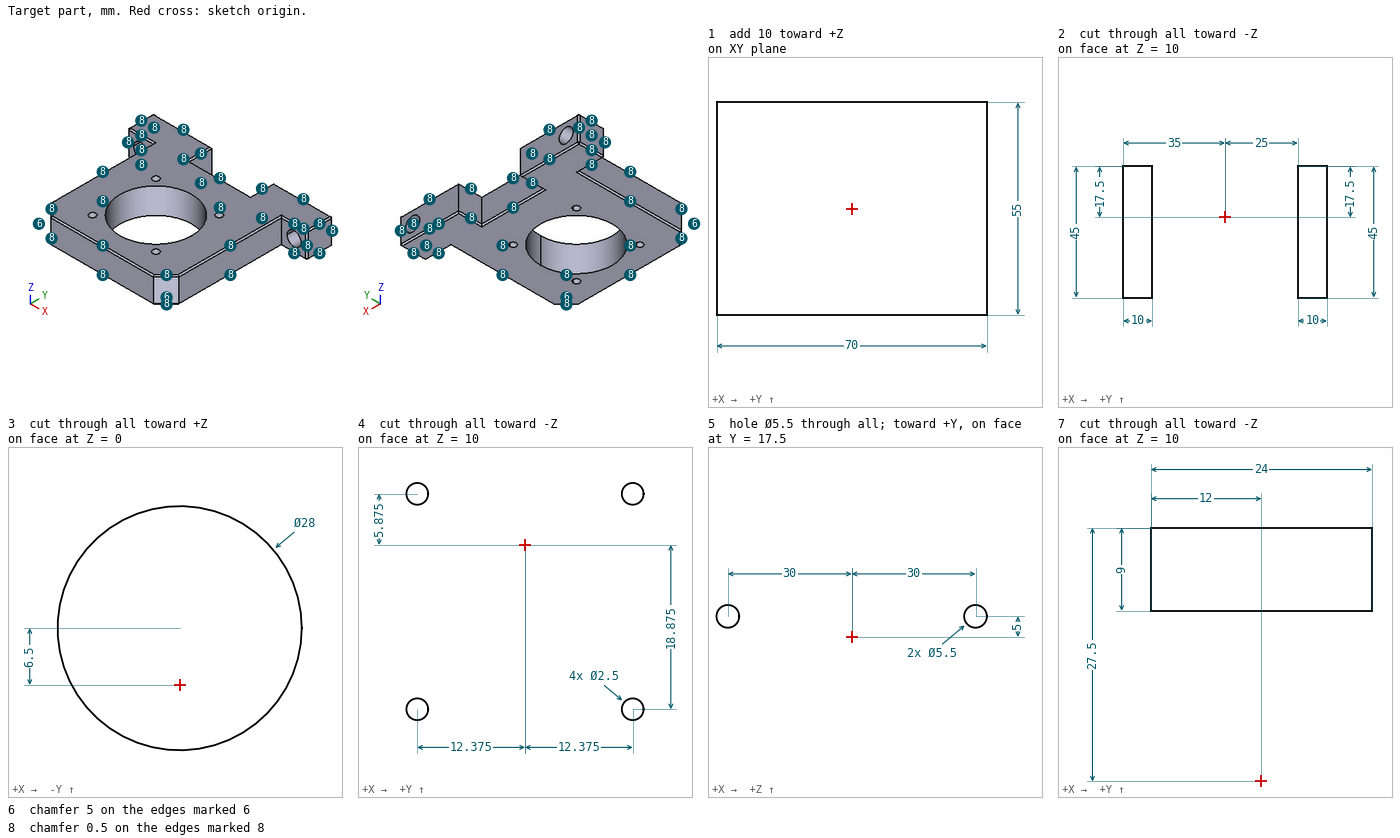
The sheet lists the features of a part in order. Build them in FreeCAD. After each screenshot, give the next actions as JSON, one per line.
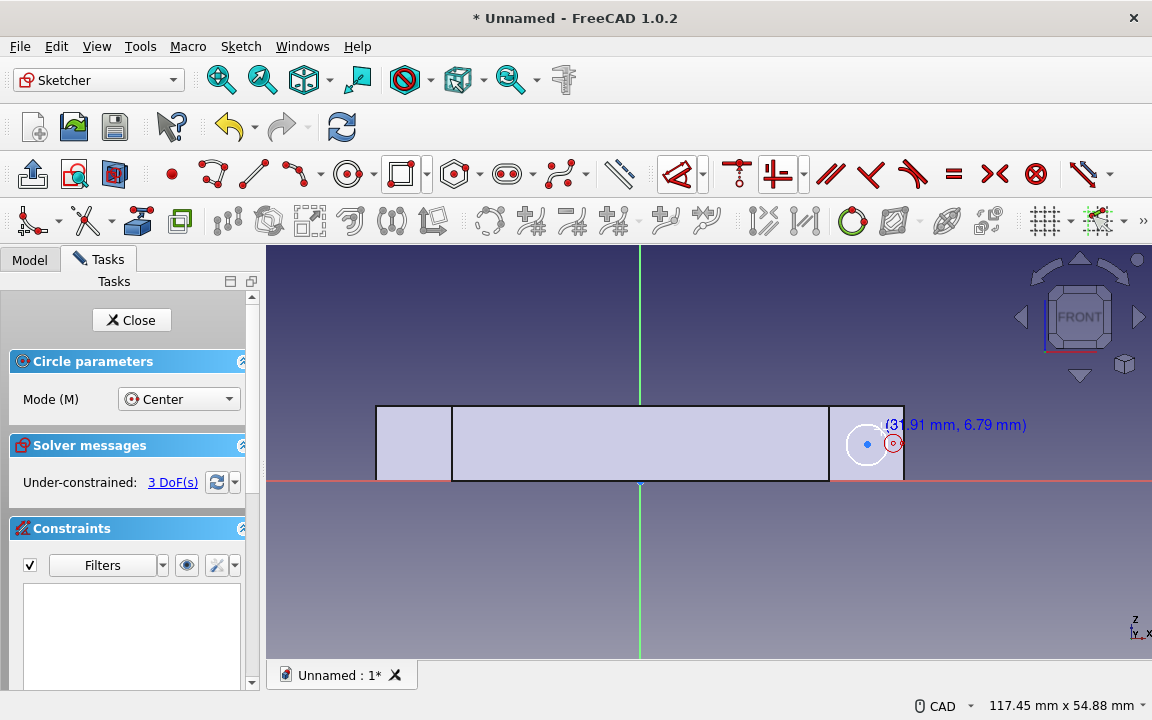
{"action": "left_click", "coordinate": [414, 444]}
{"action": "left_click", "coordinate": [429, 429]}
{"action": "key", "text": "Escape"}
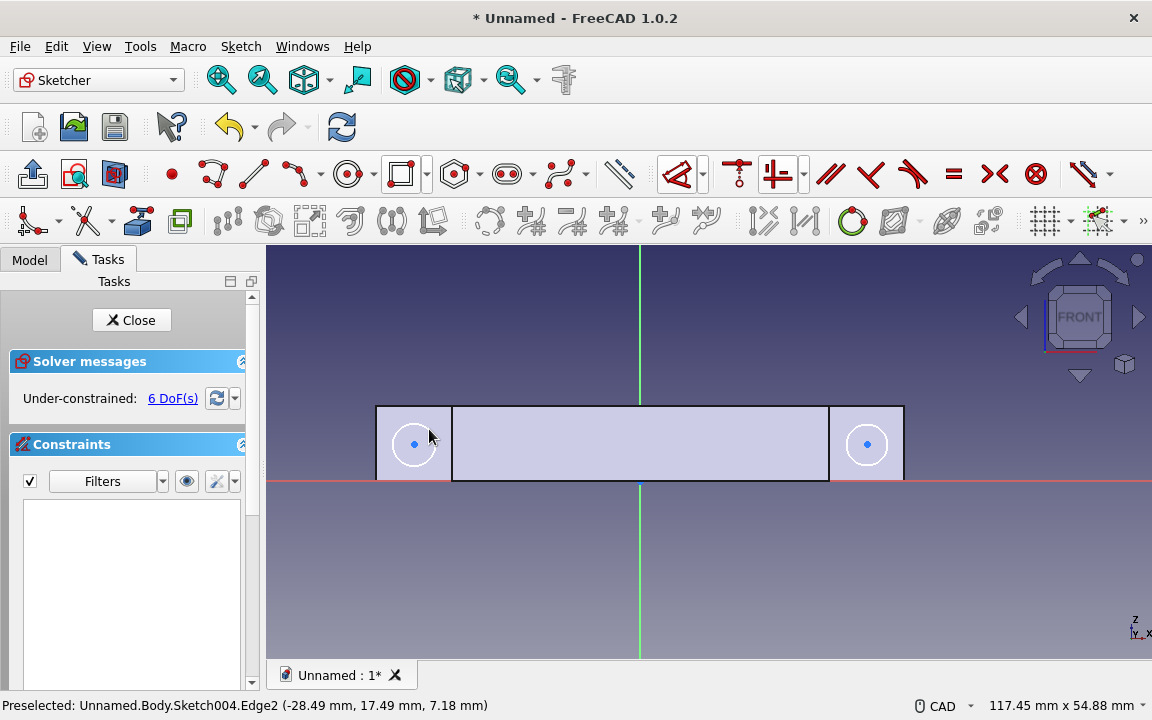
{"action": "left_click", "coordinate": [881, 430]}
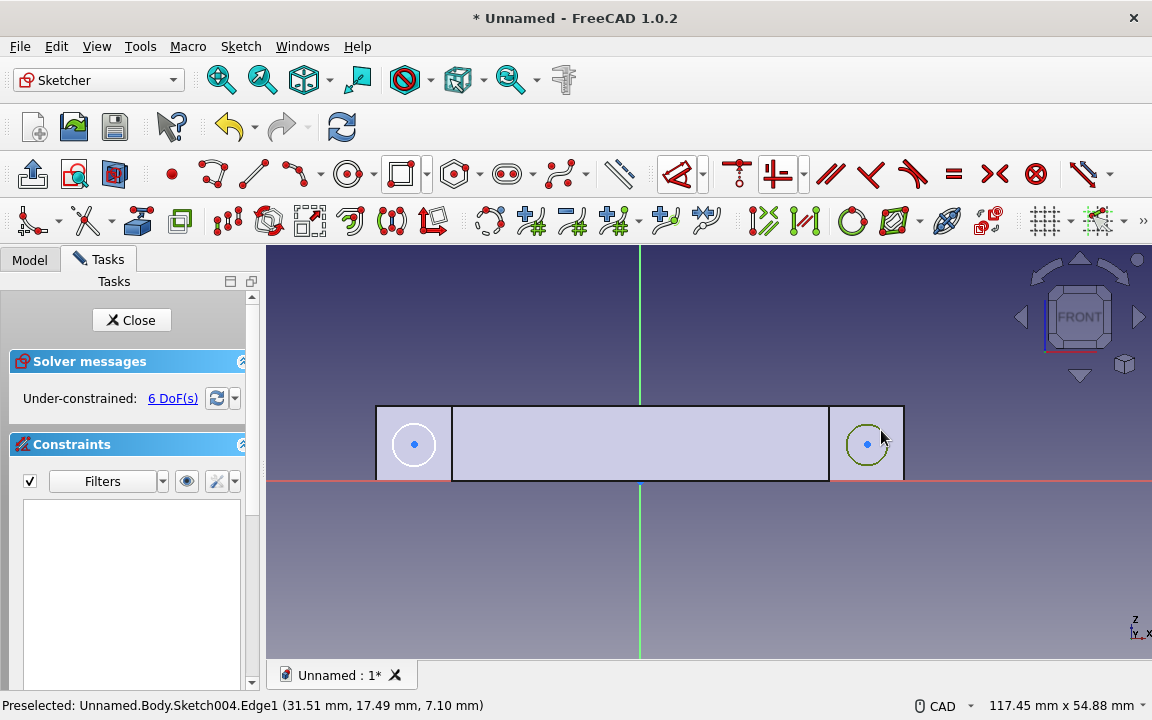
{"action": "left_click", "coordinate": [429, 430]}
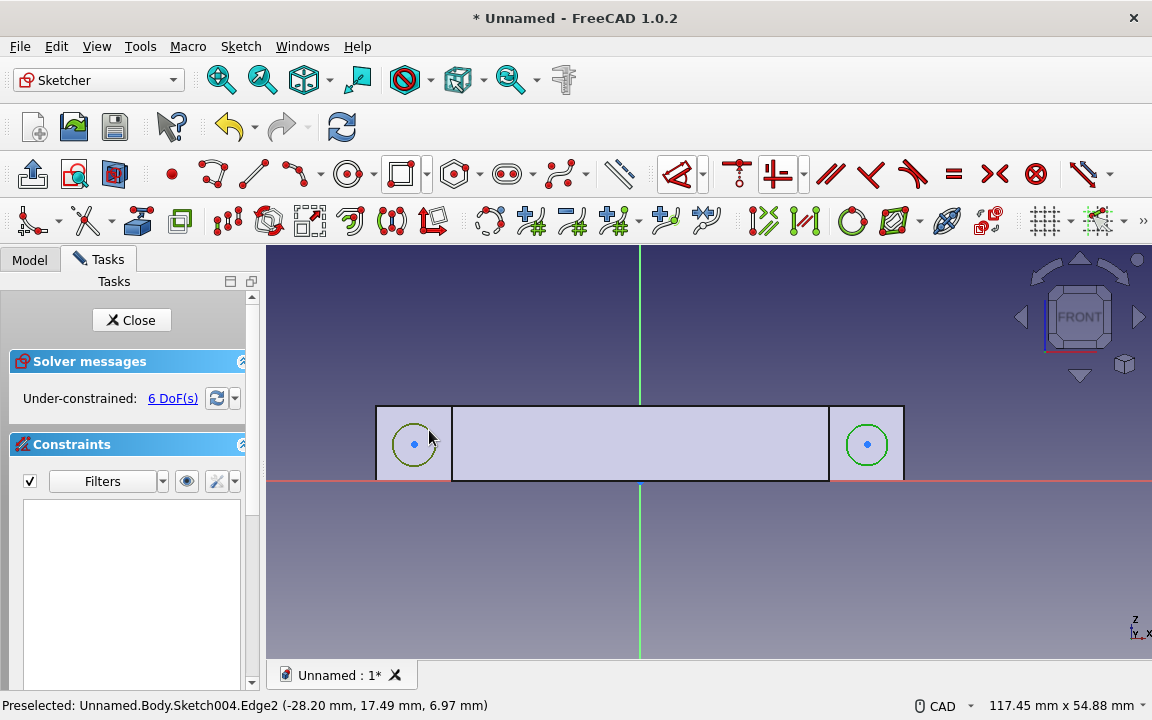
{"action": "left_click", "coordinate": [954, 174]}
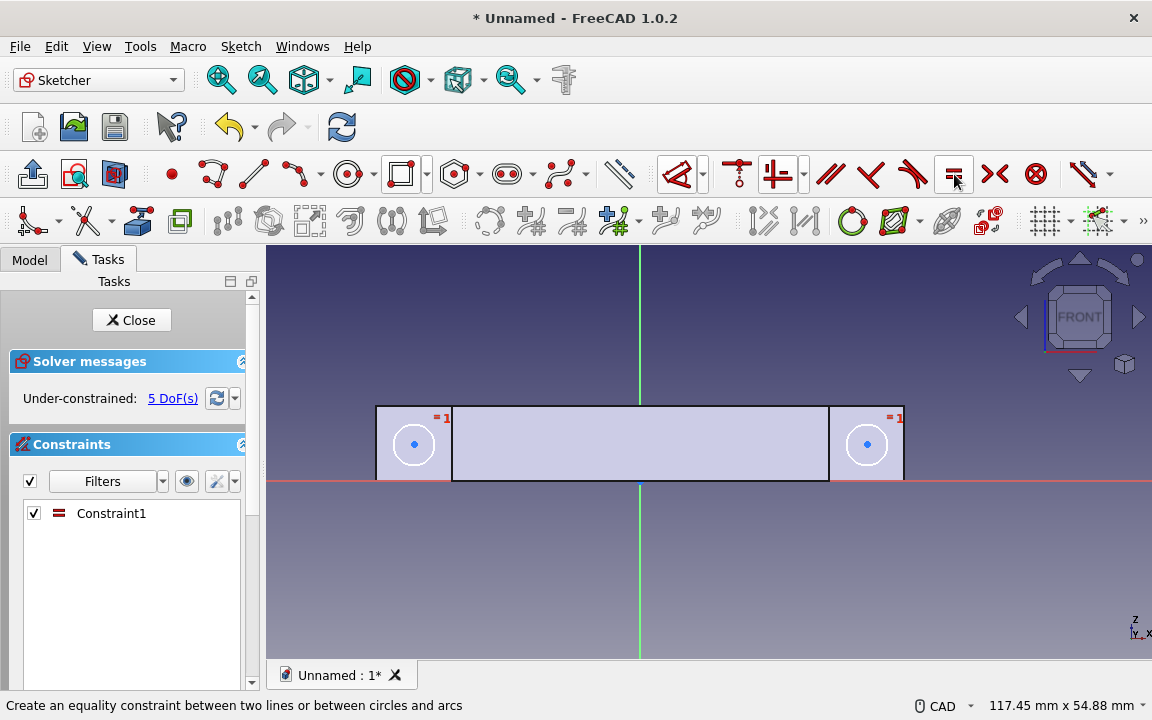
{"action": "left_click", "coordinate": [867, 445]}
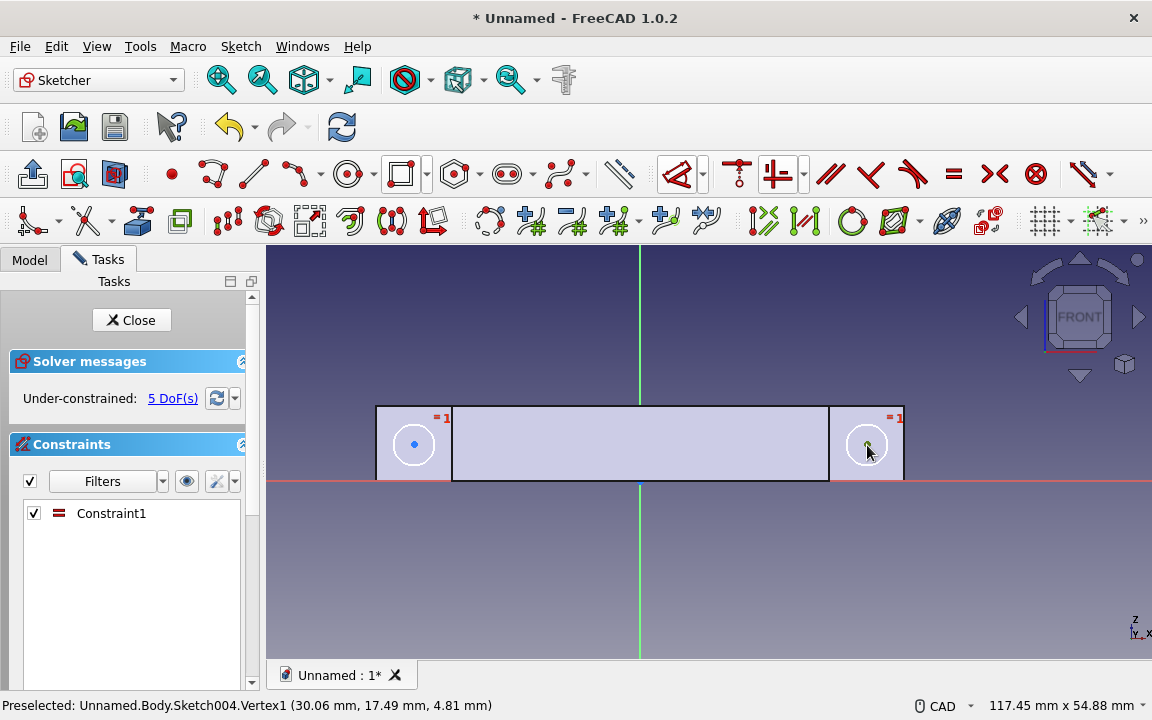
{"action": "left_click", "coordinate": [414, 445]}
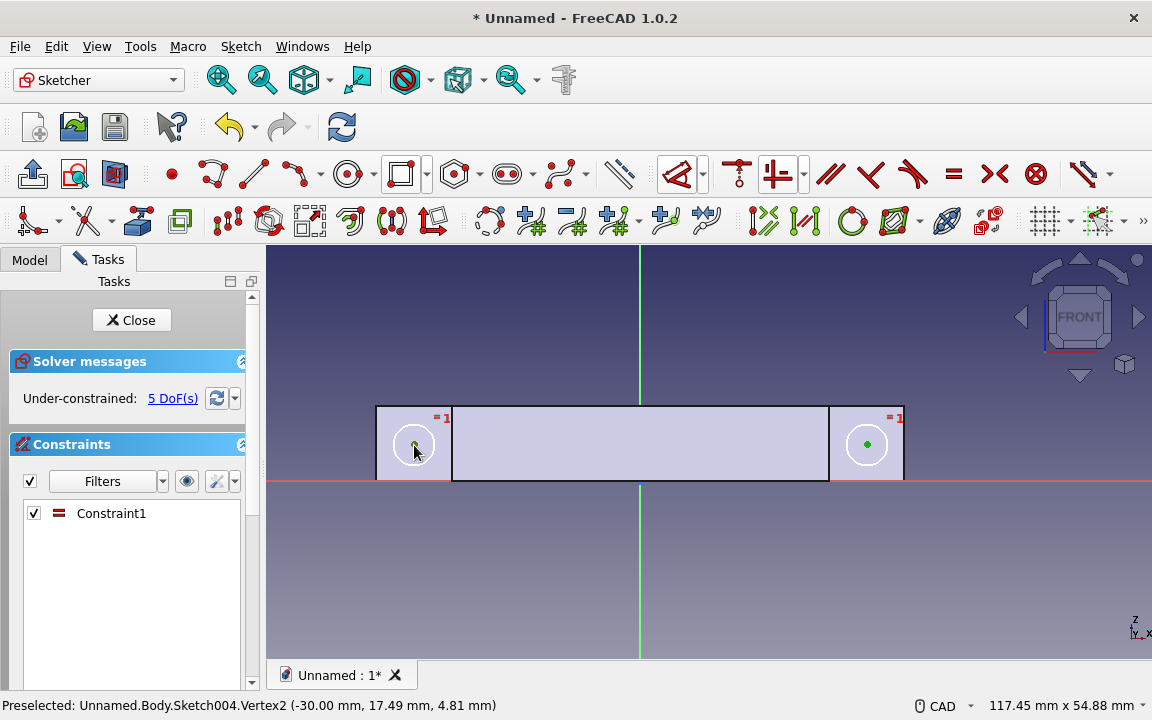
{"action": "key", "text": "h"}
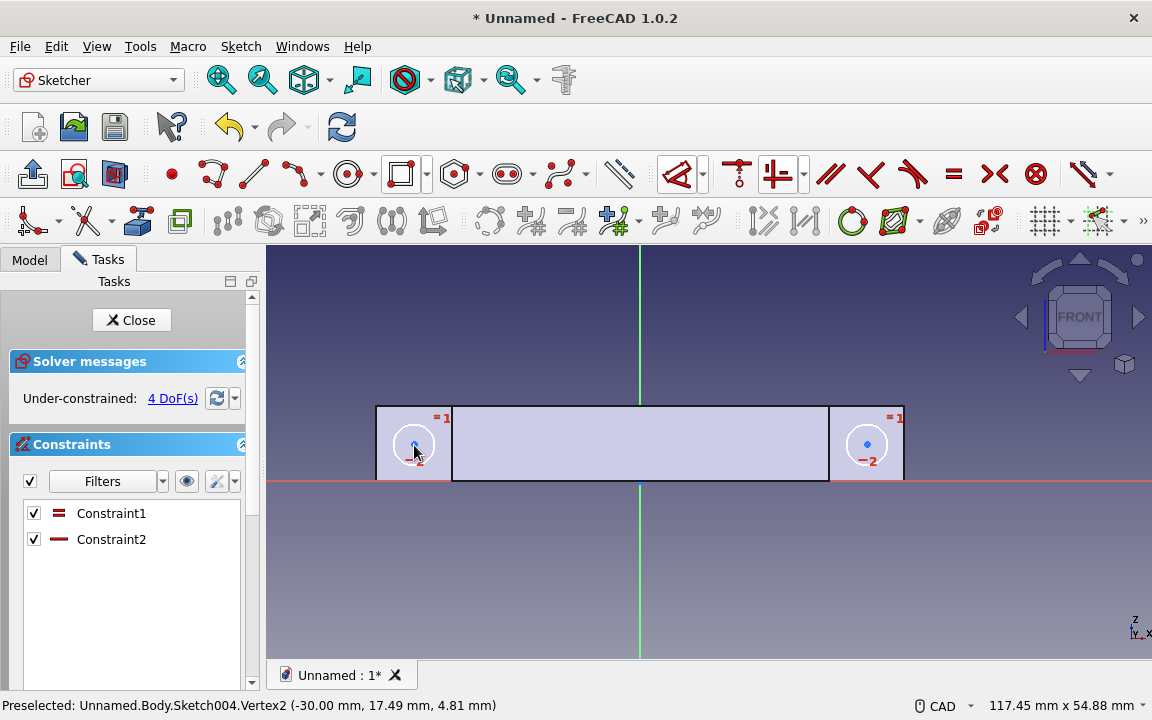
{"action": "left_click", "coordinate": [881, 430]}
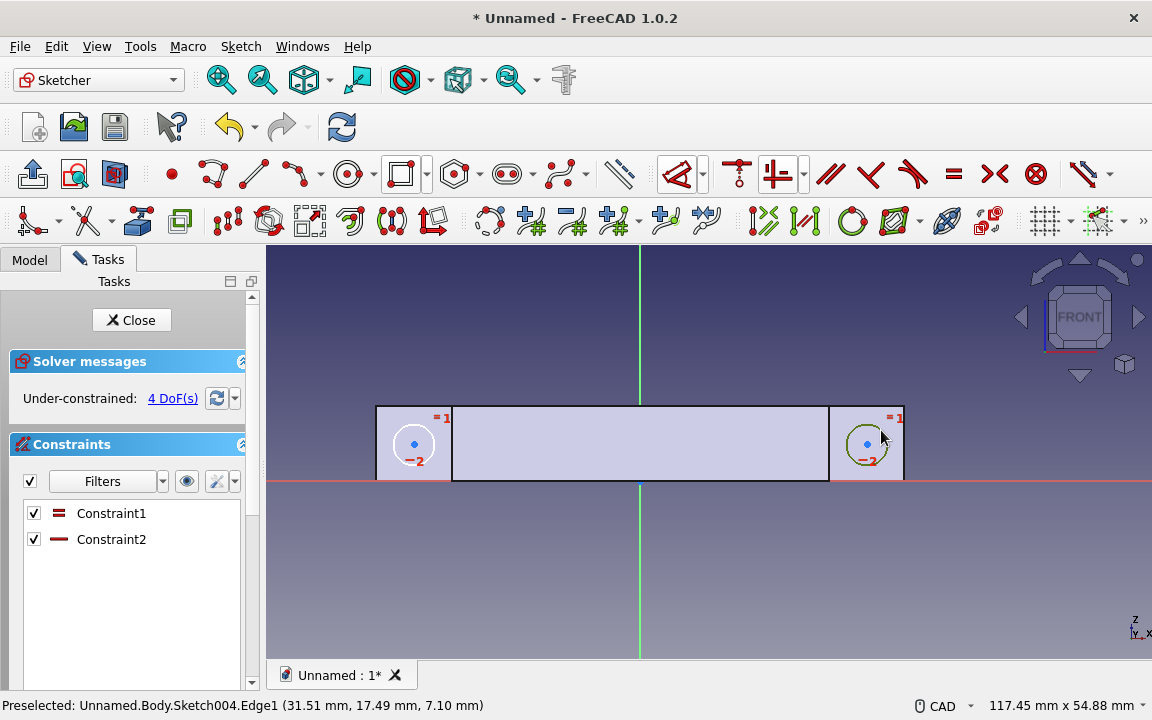
{"action": "key", "text": "k o"}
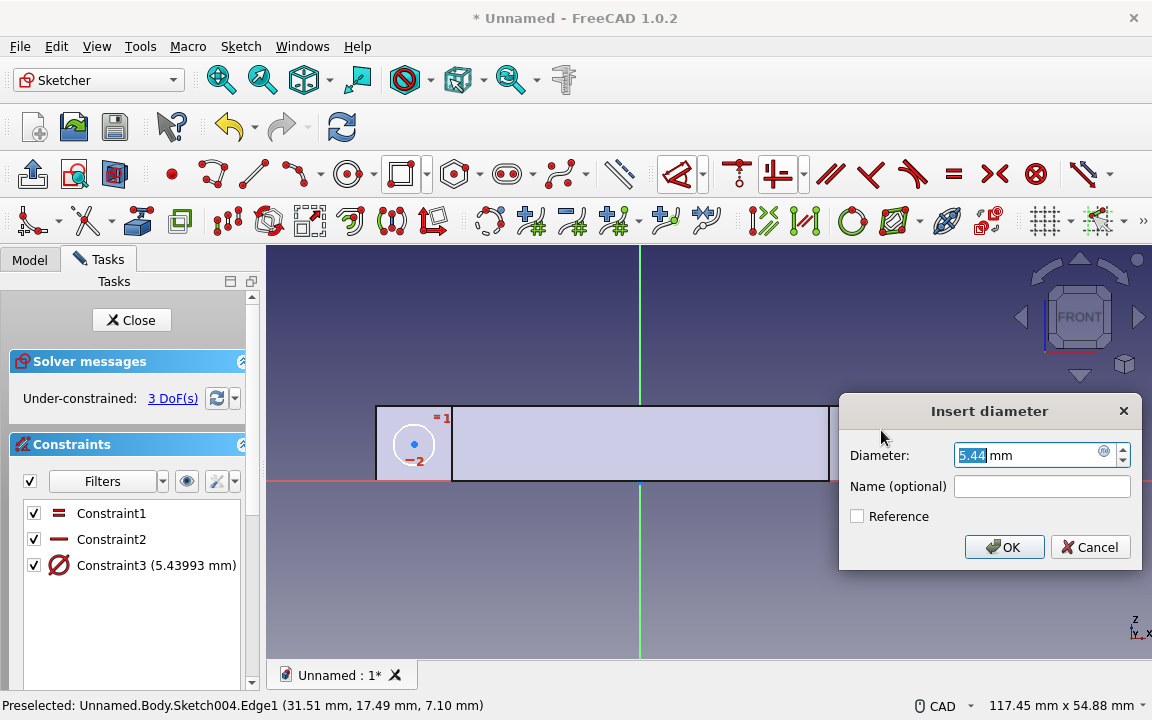
{"action": "type", "text": "5.5"}
{"action": "key", "text": "Return"}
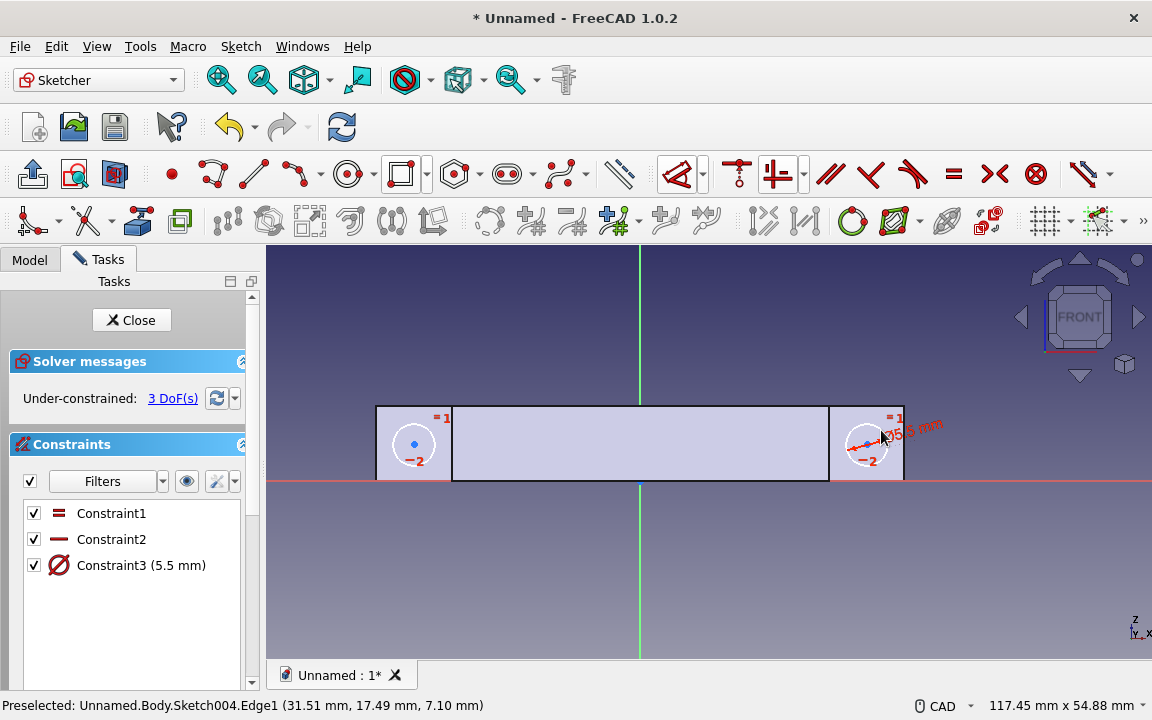
{"action": "left_click", "coordinate": [867, 445]}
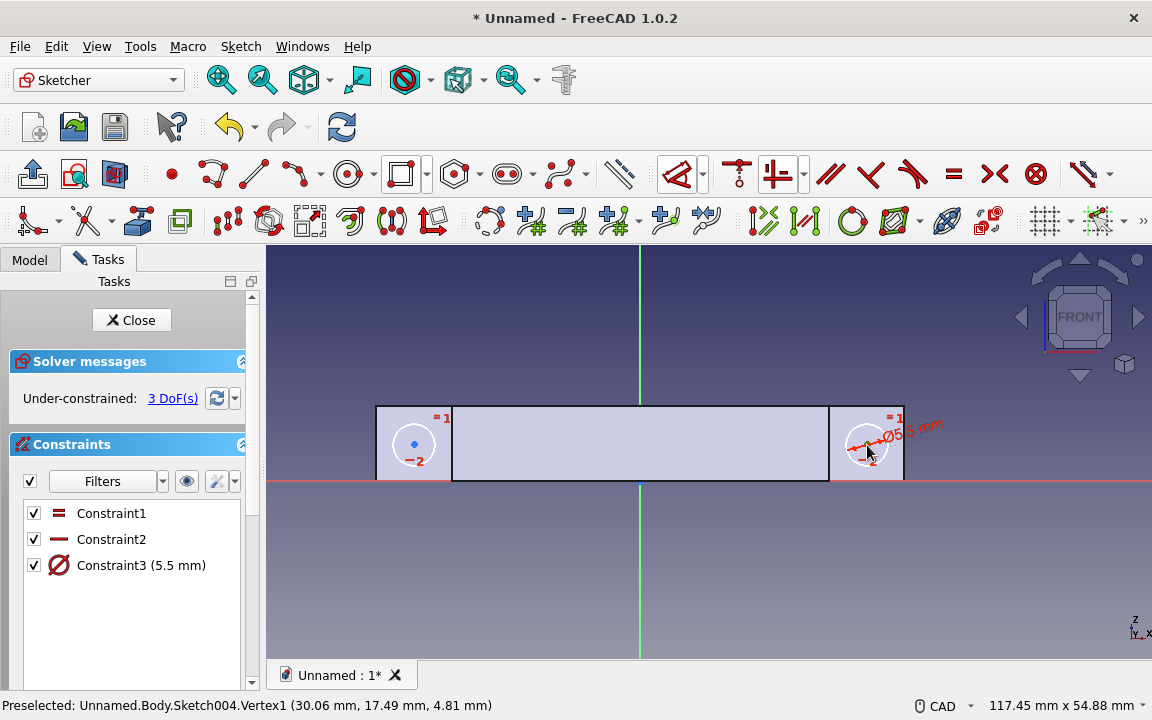
{"action": "left_click", "coordinate": [702, 174]}